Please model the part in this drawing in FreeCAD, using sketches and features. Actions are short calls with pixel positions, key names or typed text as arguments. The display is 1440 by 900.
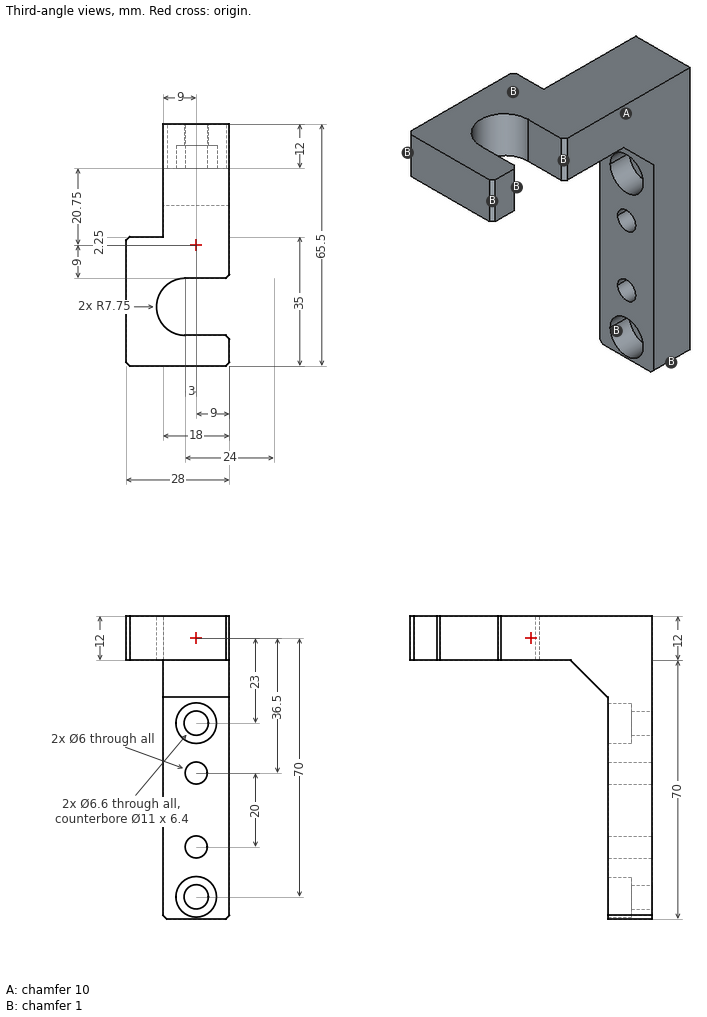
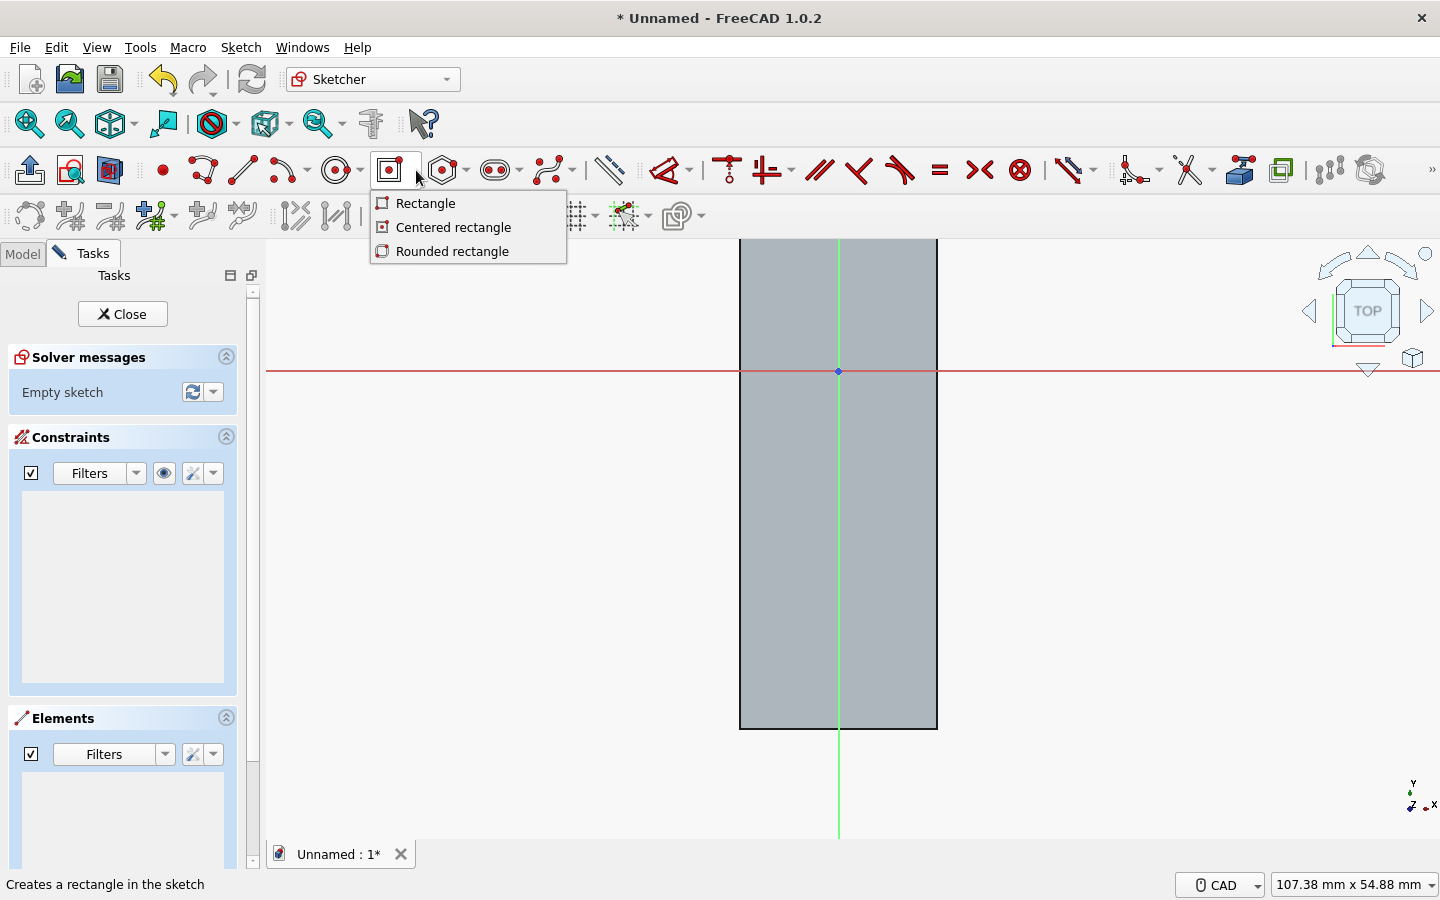
click(468, 203)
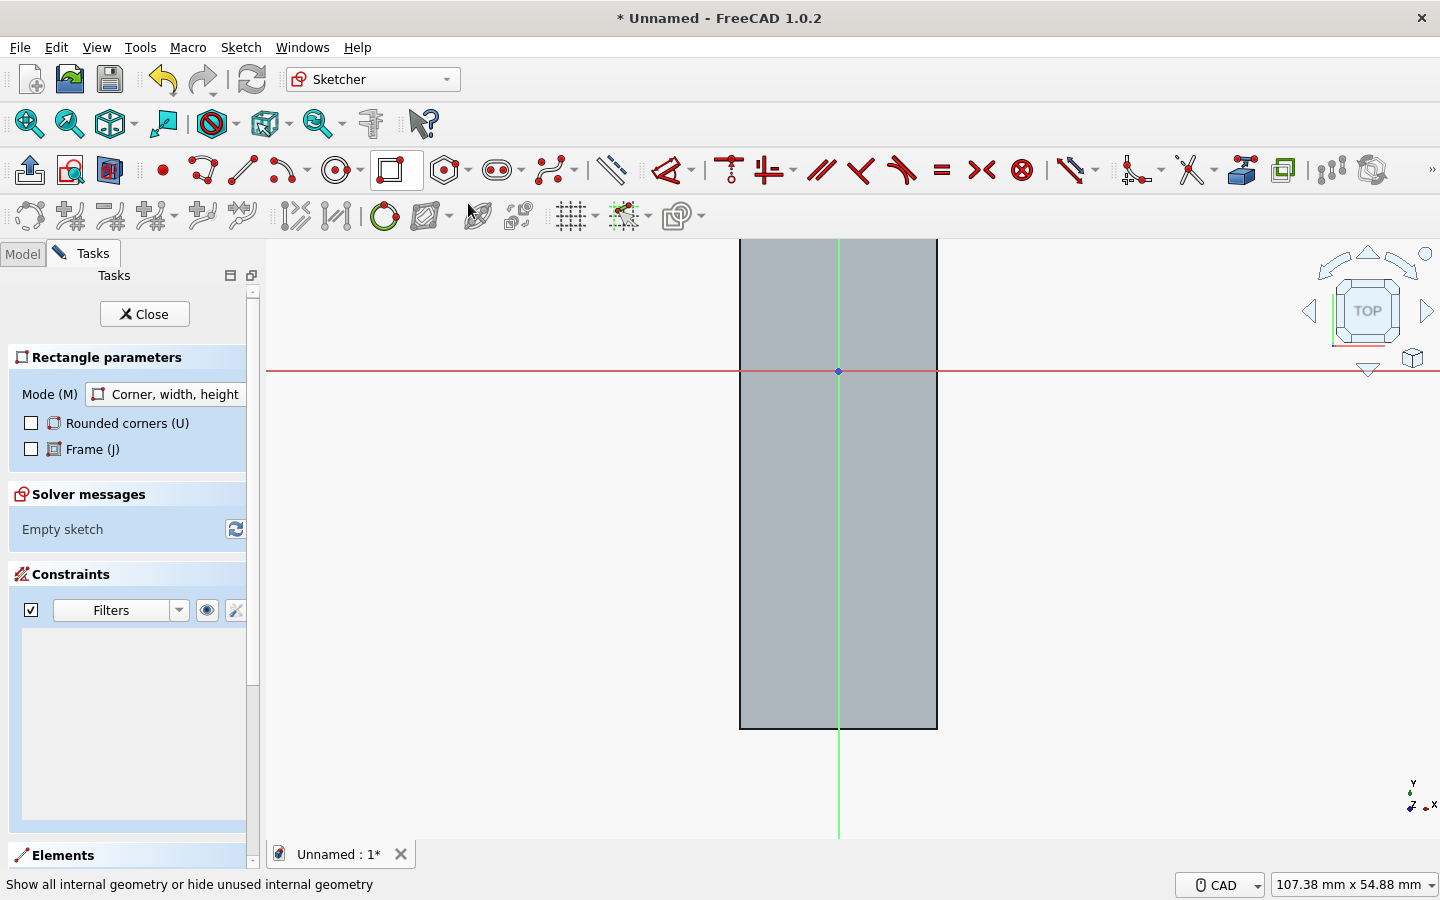
click(631, 347)
move(937, 729)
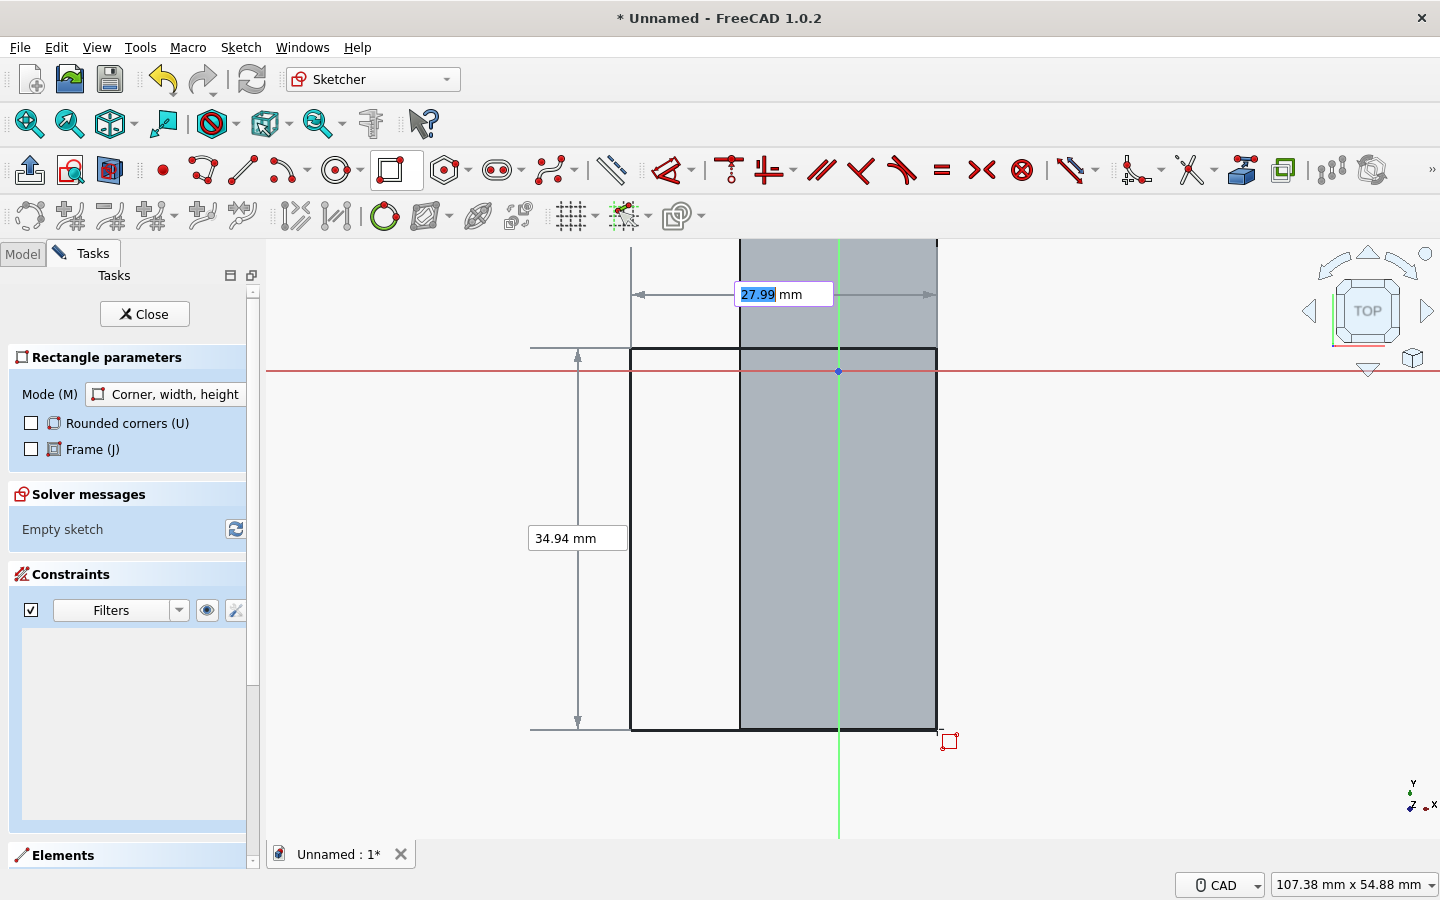
text(28)
key(Tab)
text(35)
key(Return)
key(Escape)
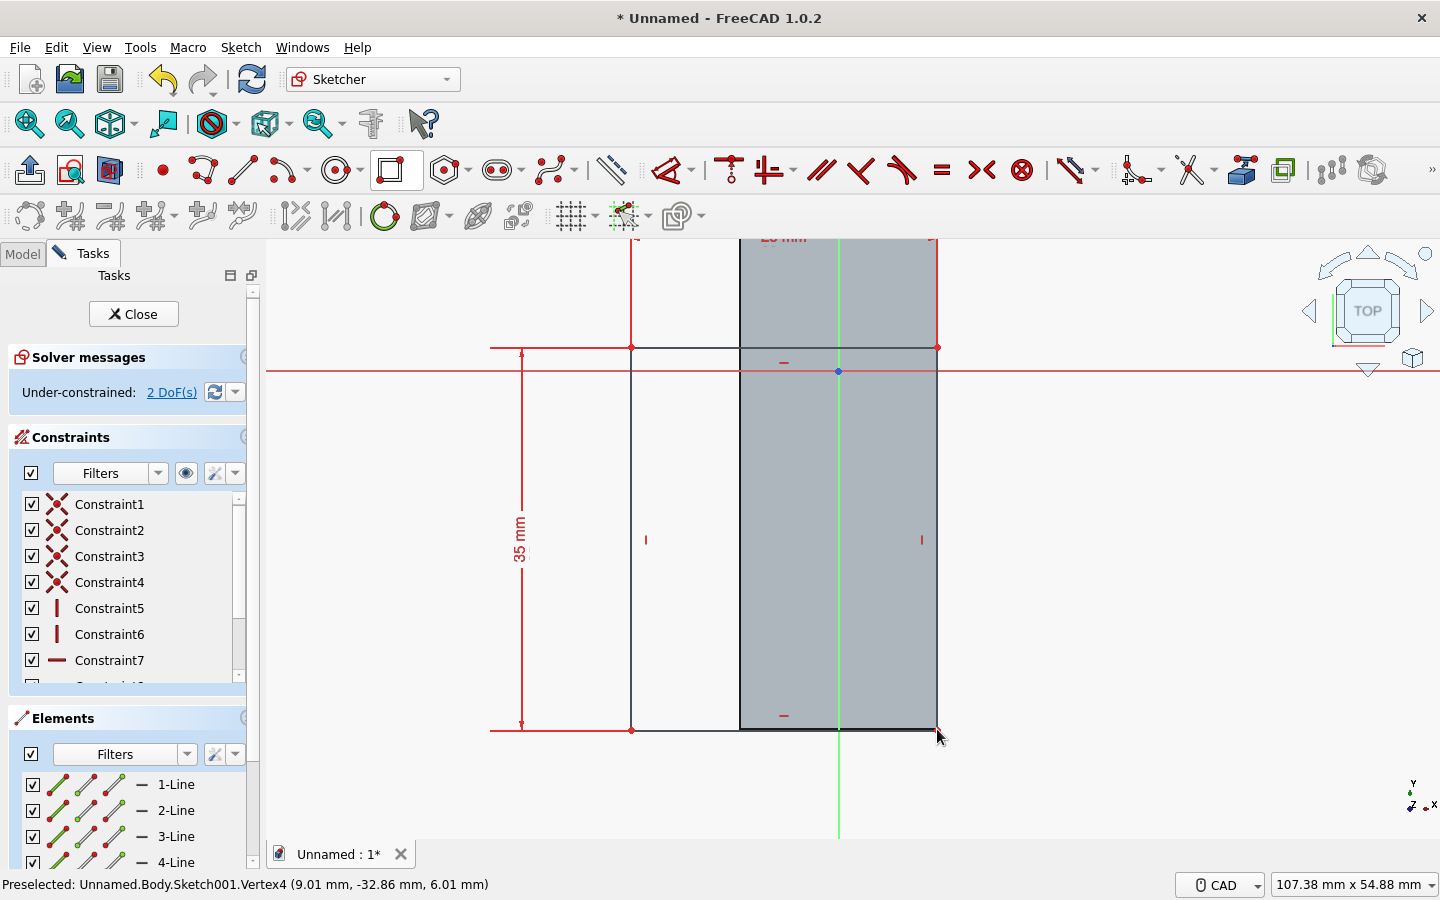
click(666, 170)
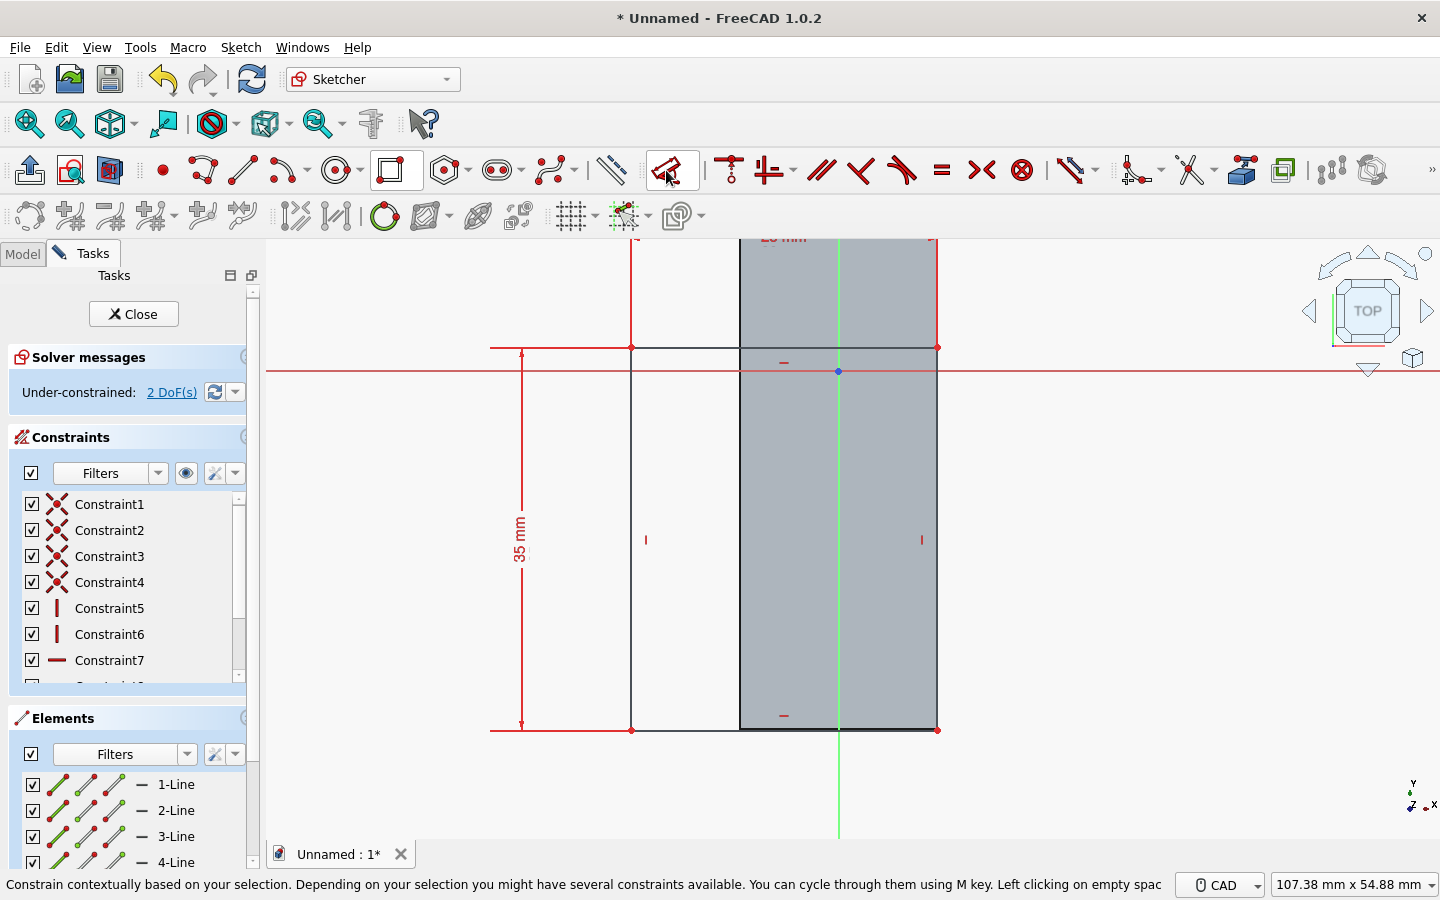
click(937, 731)
click(888, 765)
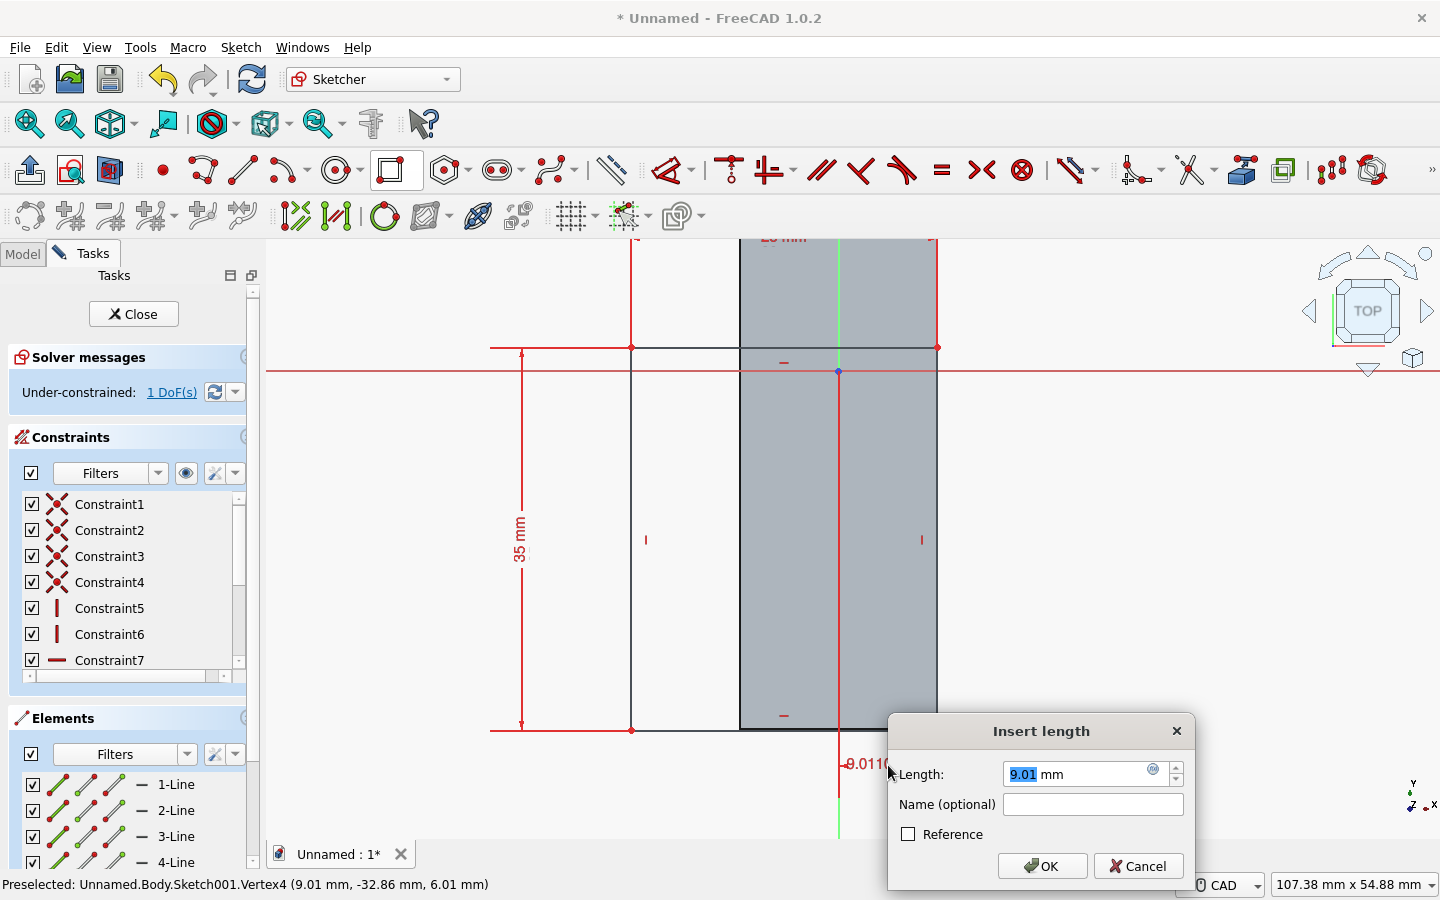
text(9)
key(Return)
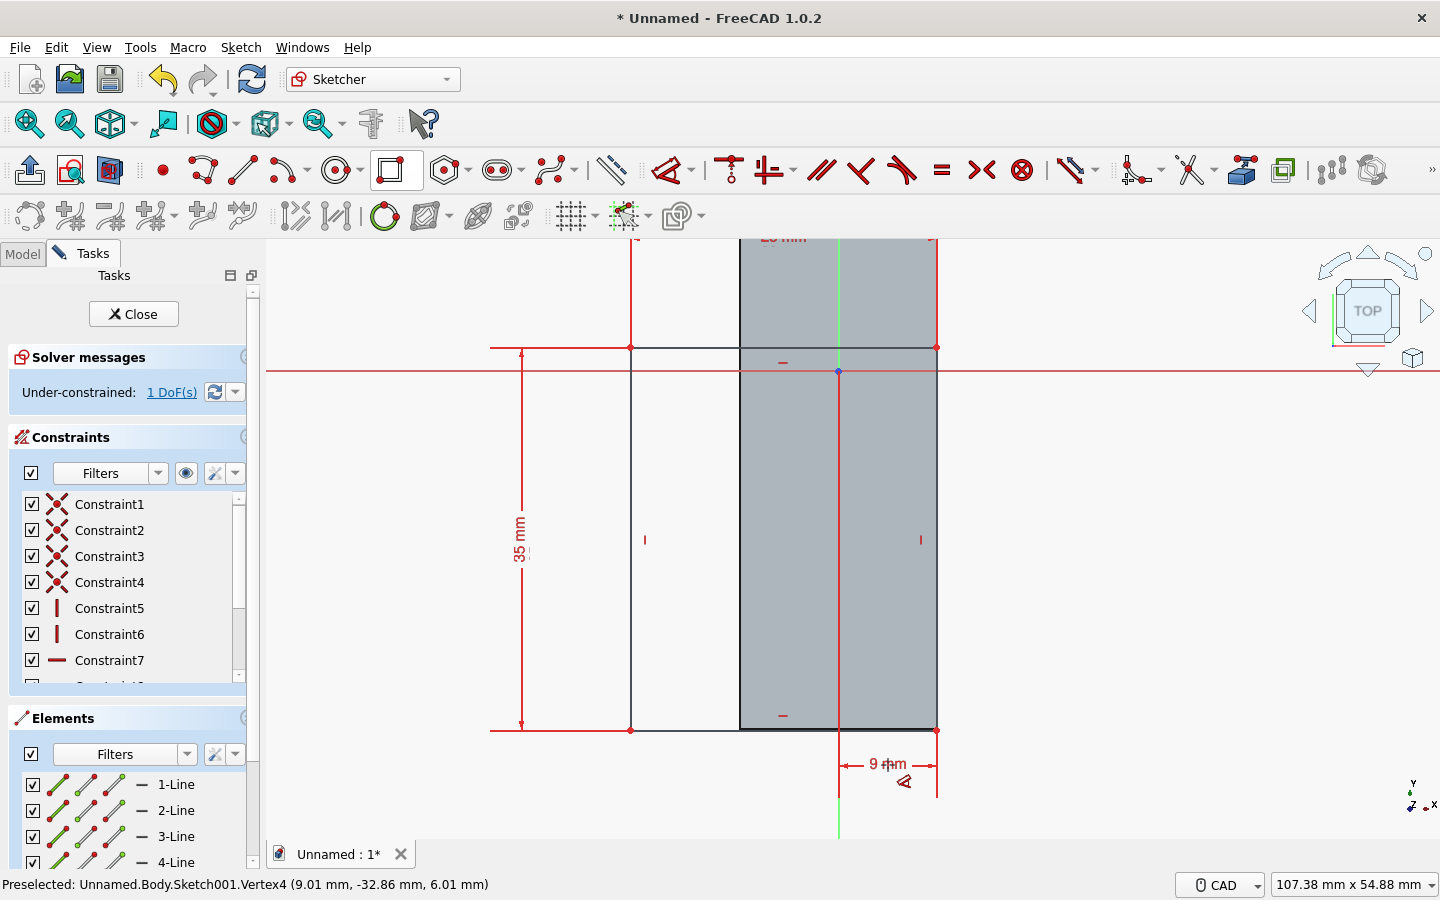
scroll(631, 348, up, 3)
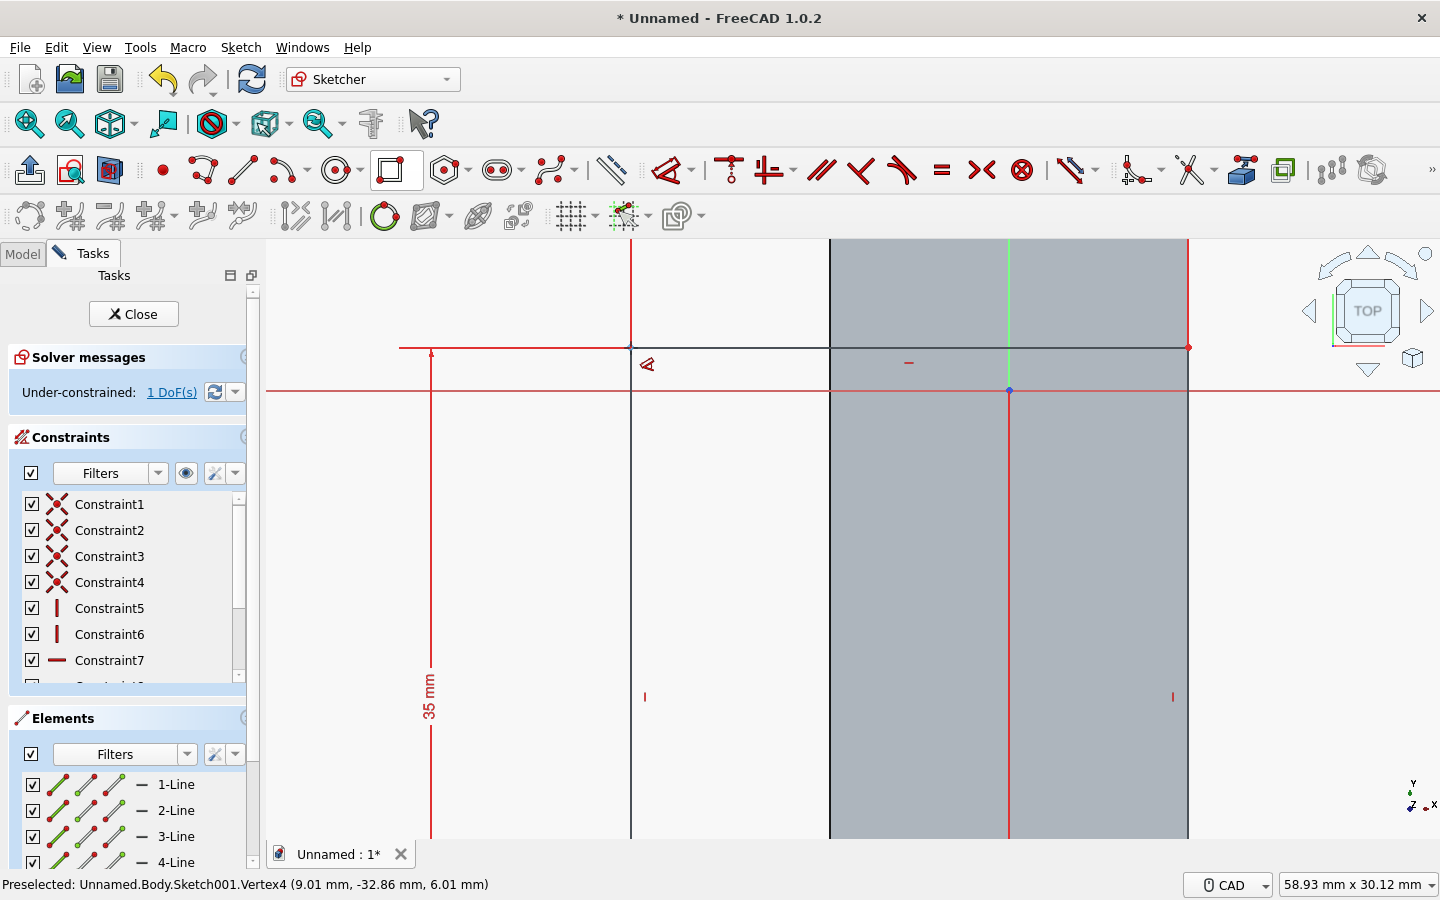
click(631, 348)
click(597, 369)